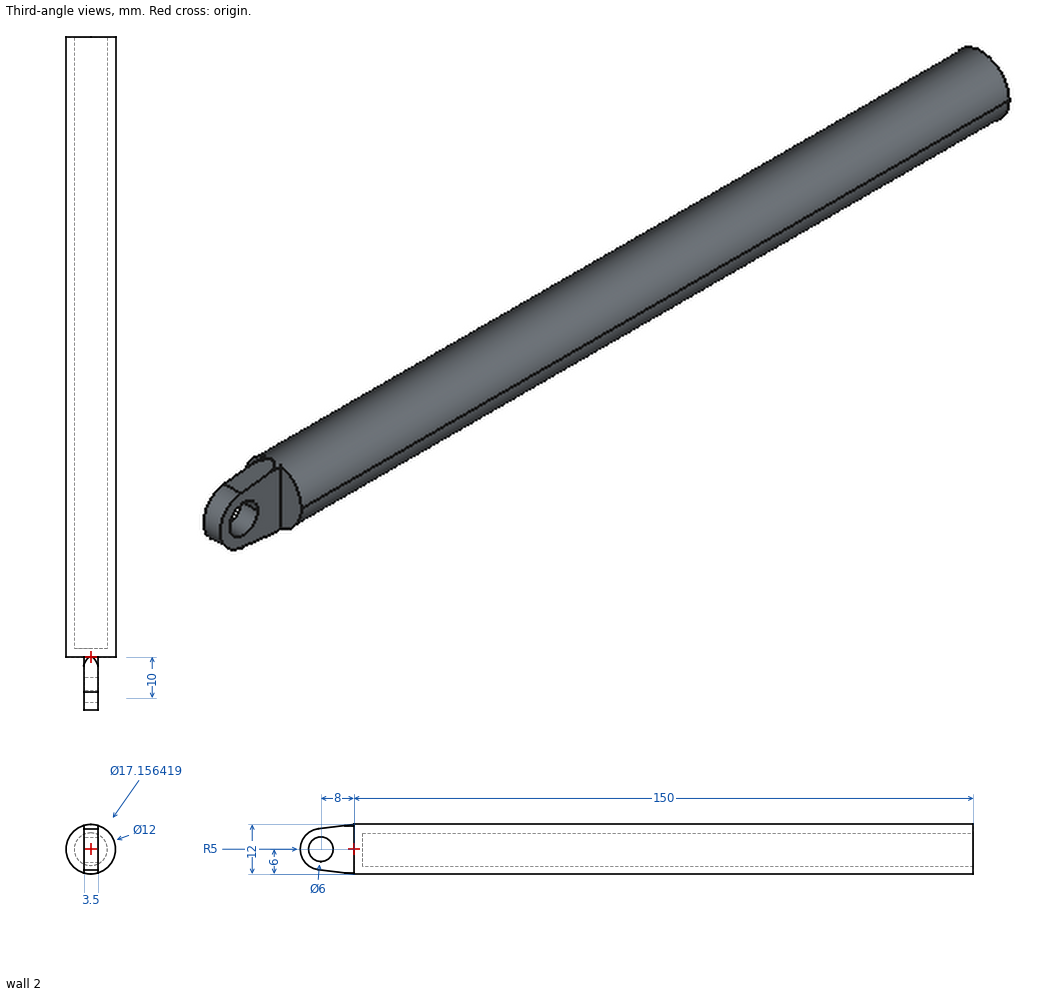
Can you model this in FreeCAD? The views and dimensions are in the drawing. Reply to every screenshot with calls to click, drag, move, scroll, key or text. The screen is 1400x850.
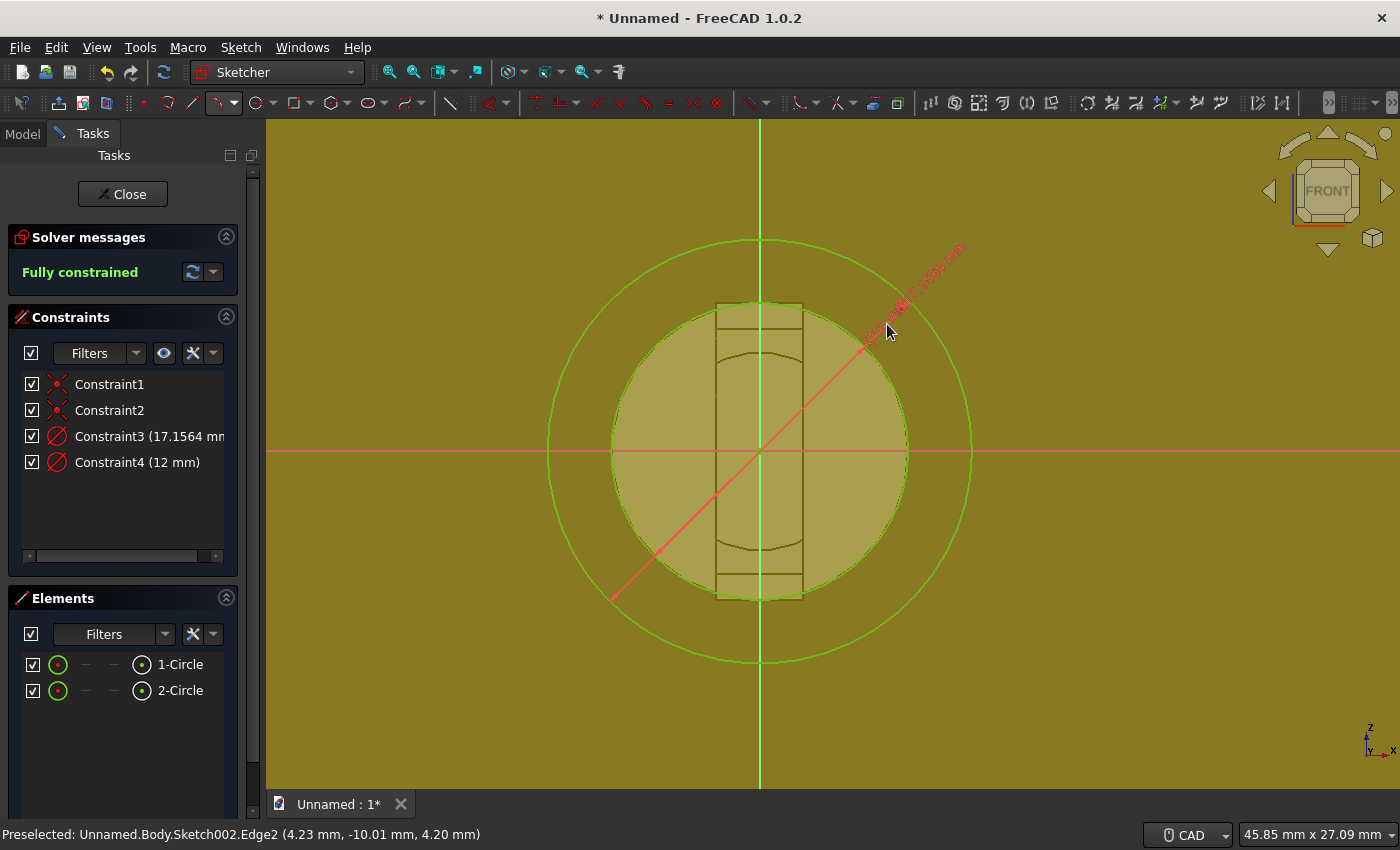
click(123, 194)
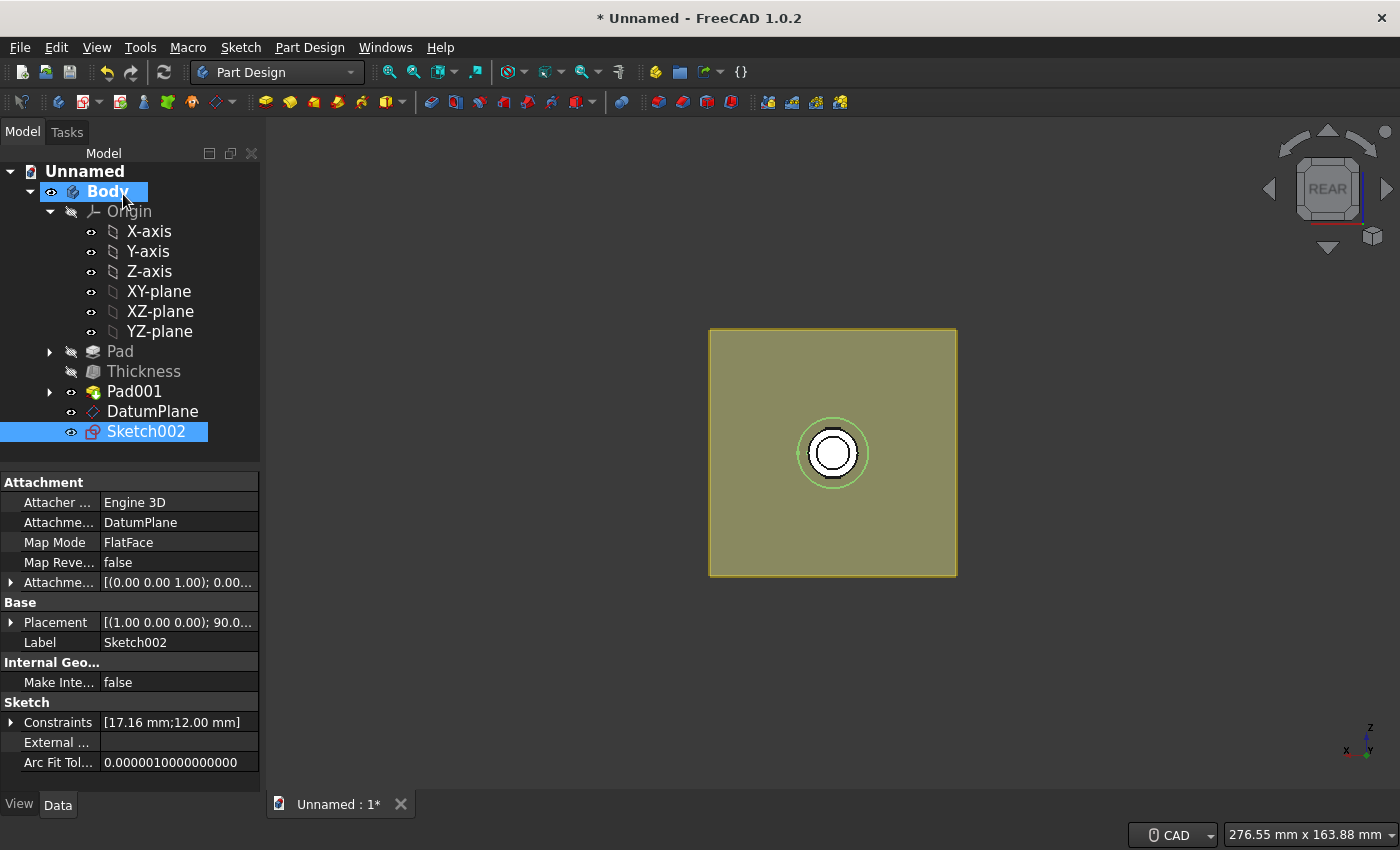
click(432, 102)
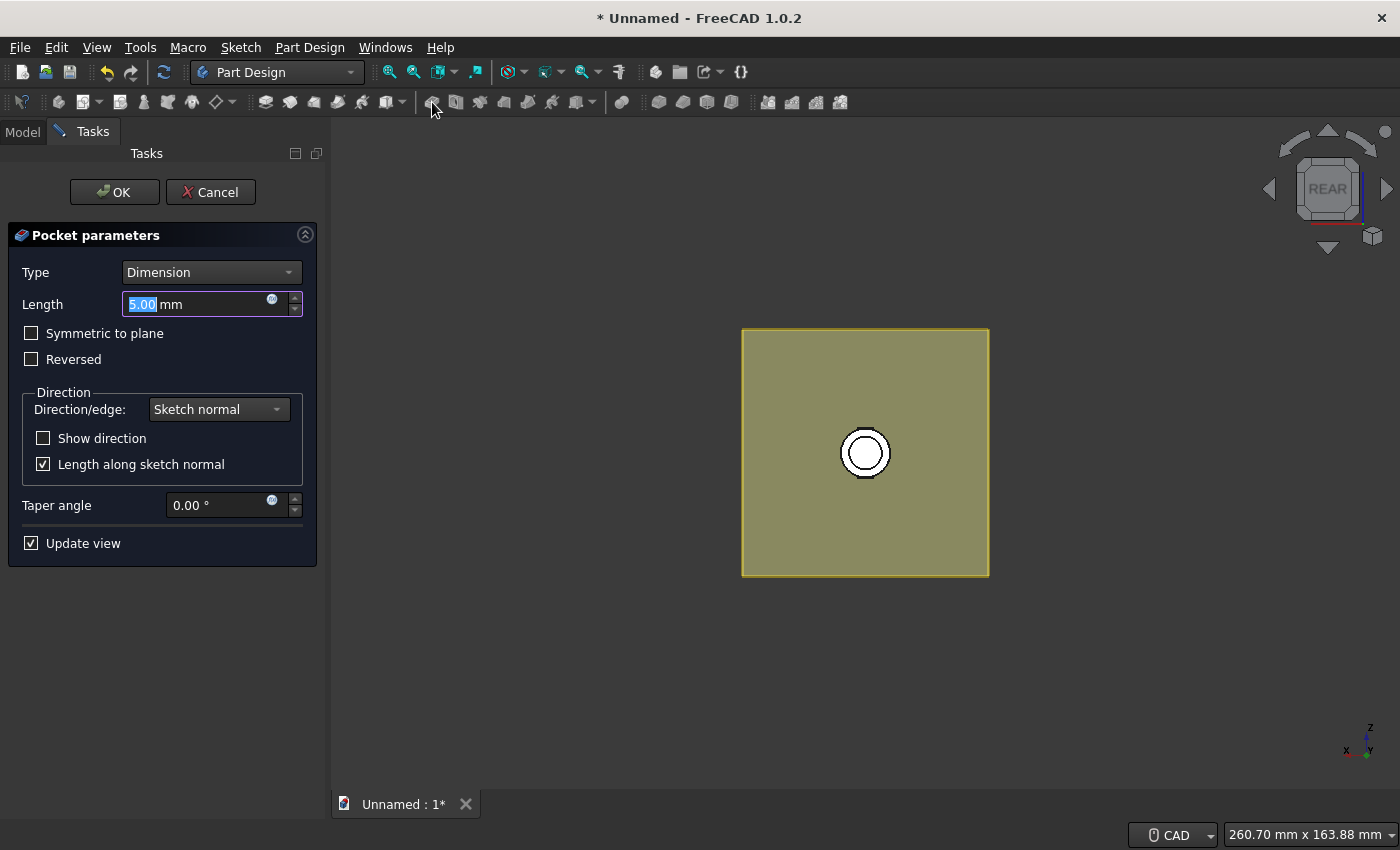
text(10)
key(Tab)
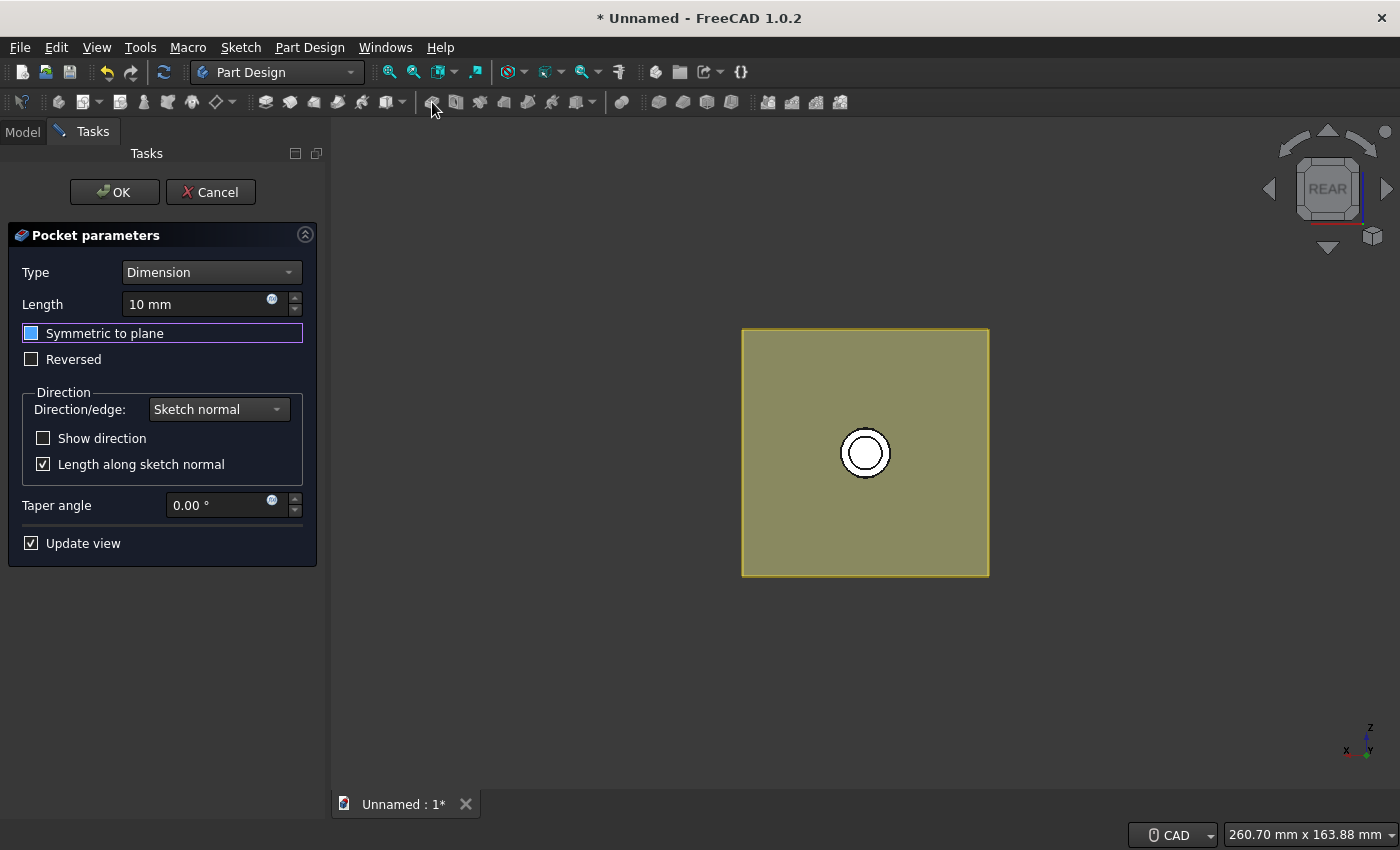
click(115, 192)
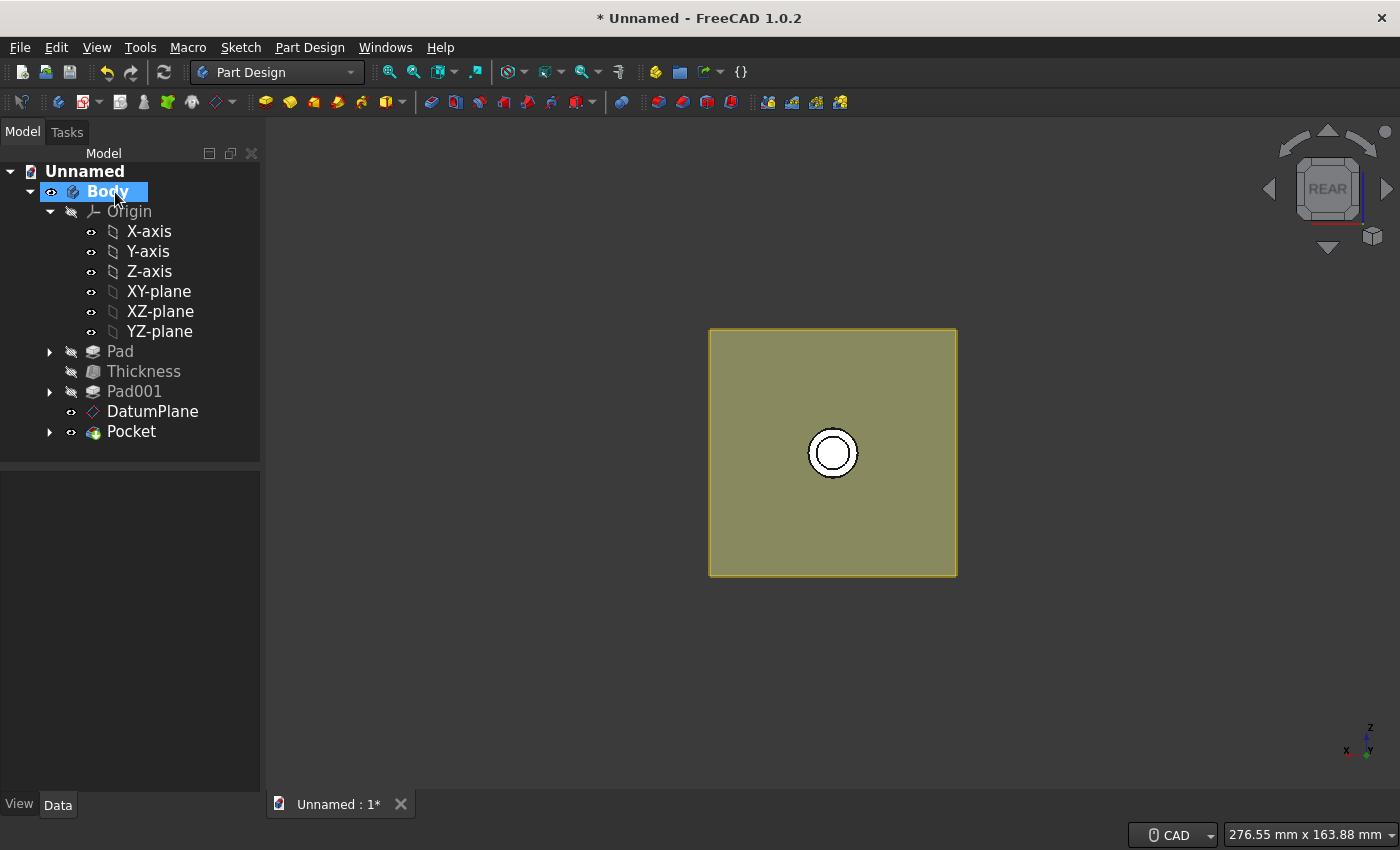
click(116, 412)
key(space)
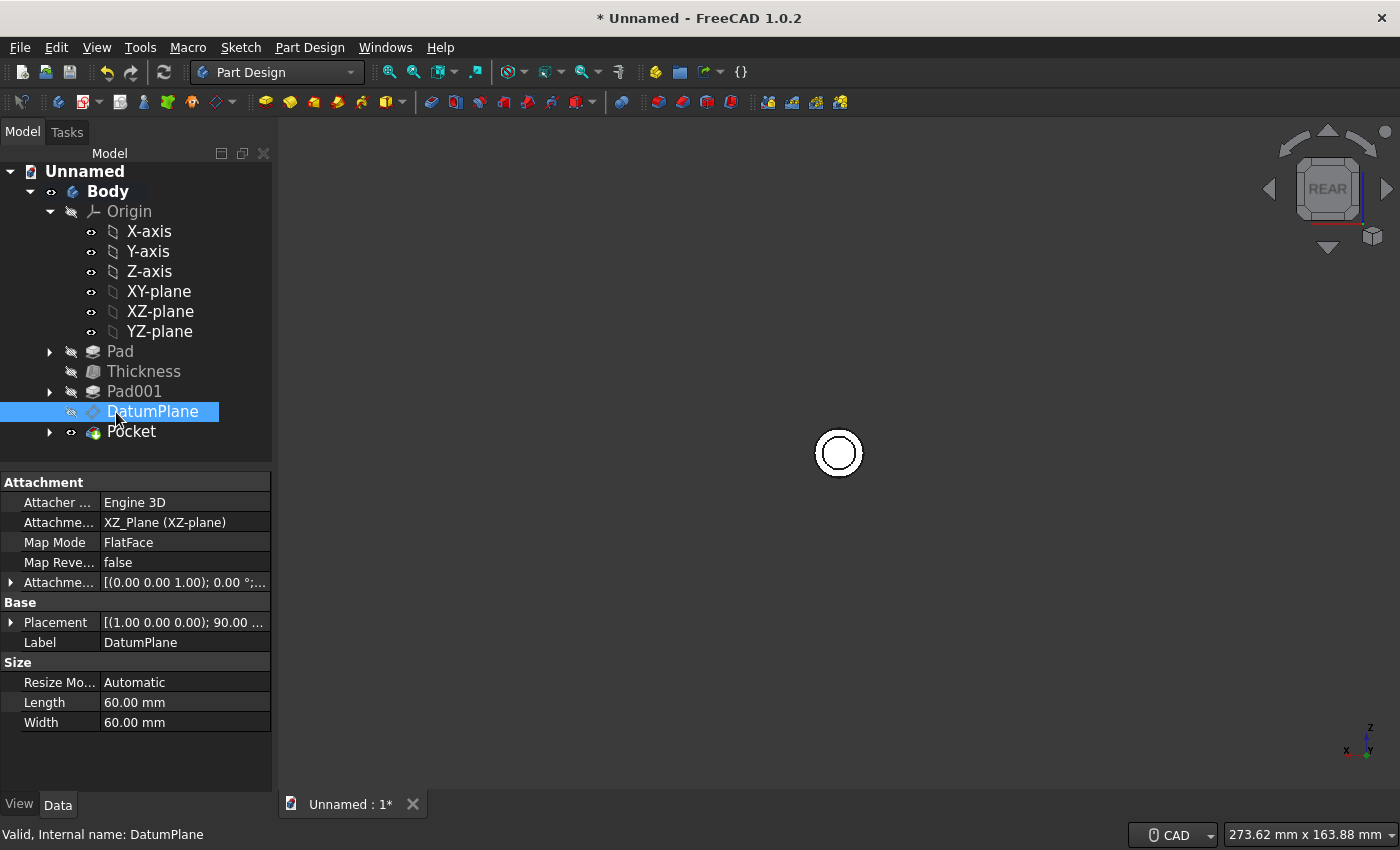
key(0)